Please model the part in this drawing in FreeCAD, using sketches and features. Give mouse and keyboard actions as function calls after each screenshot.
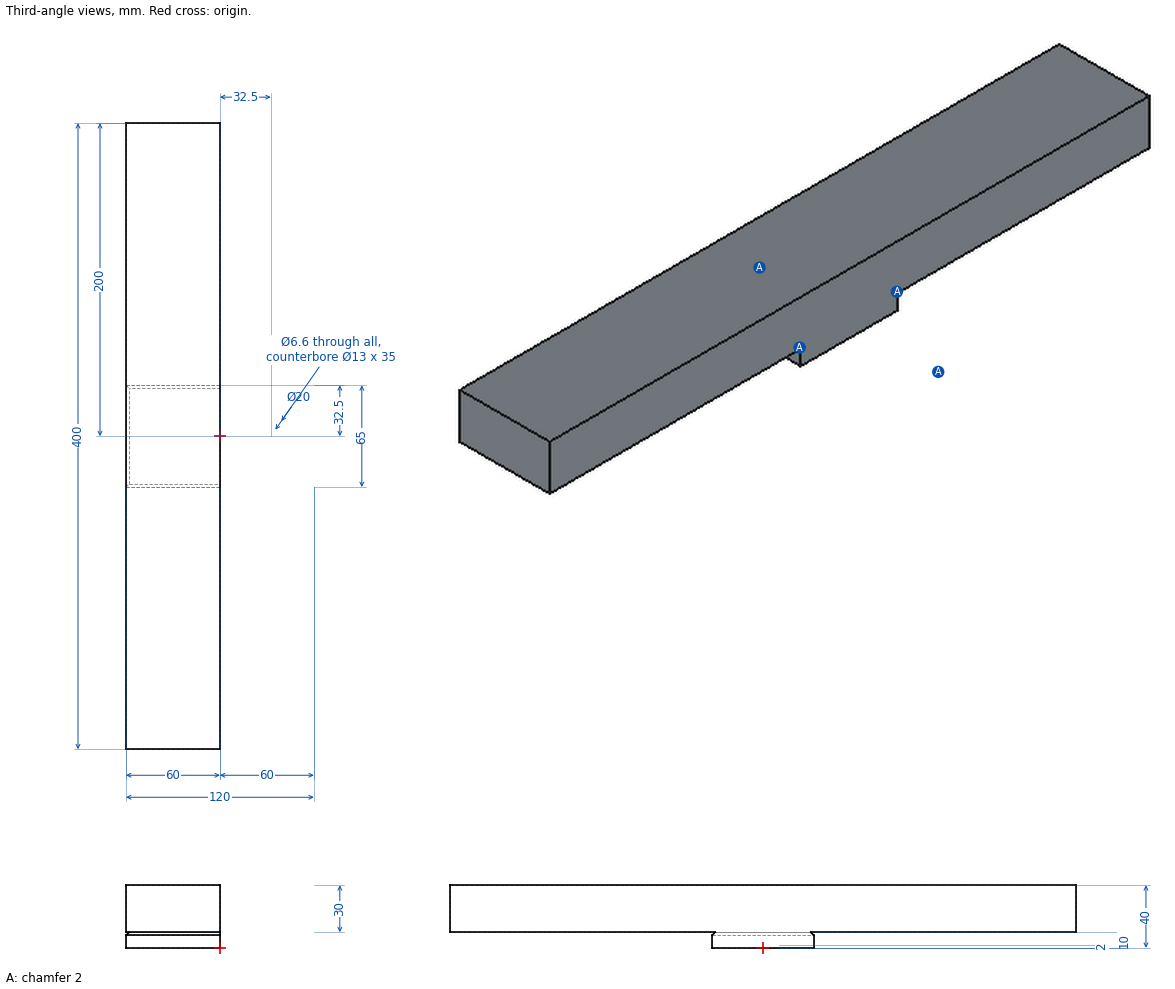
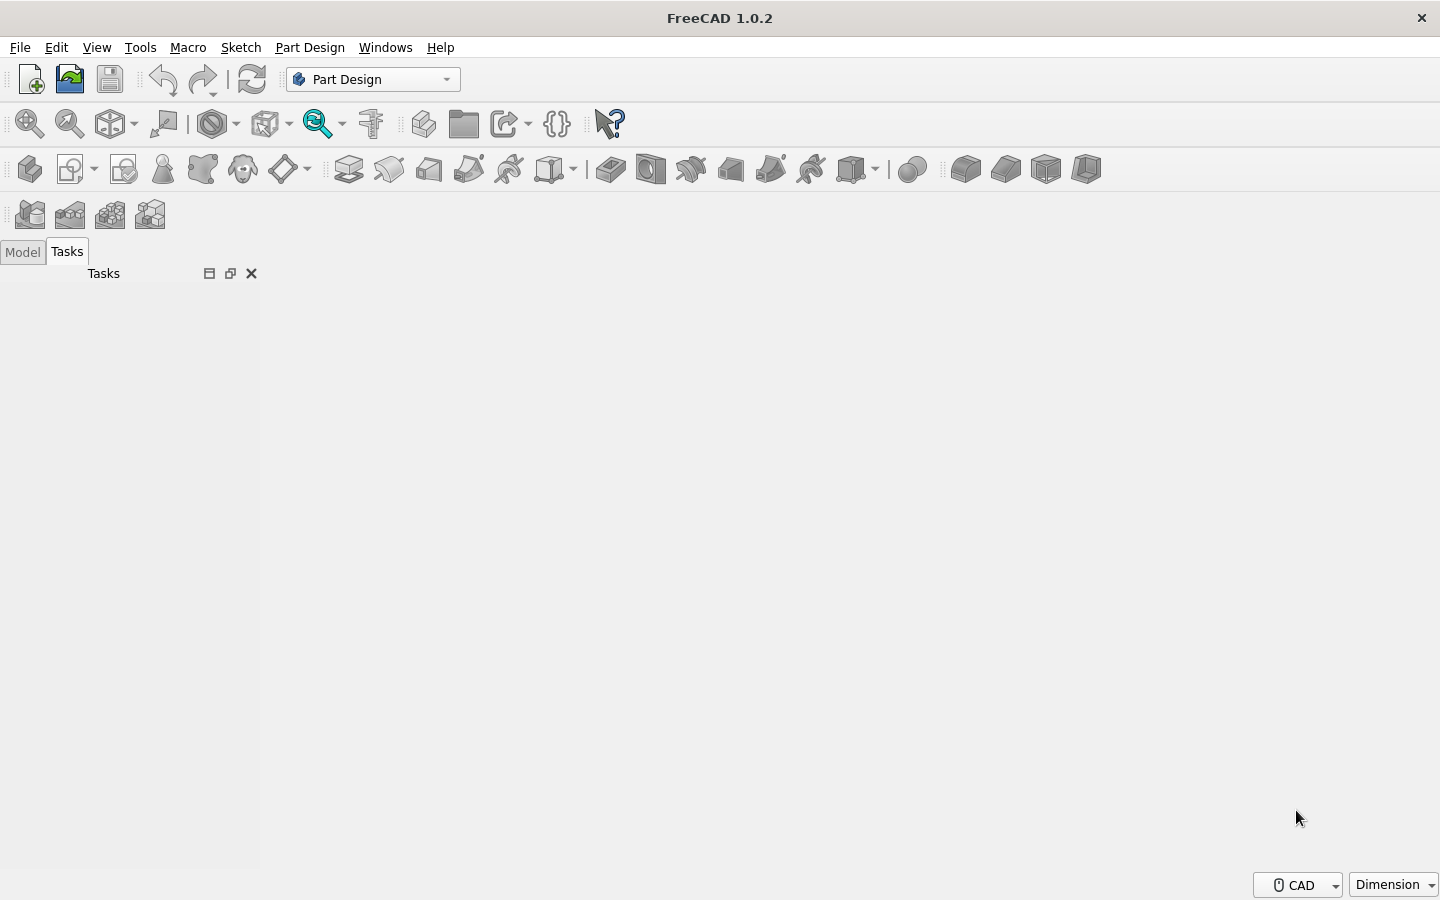
key(ctrl+n)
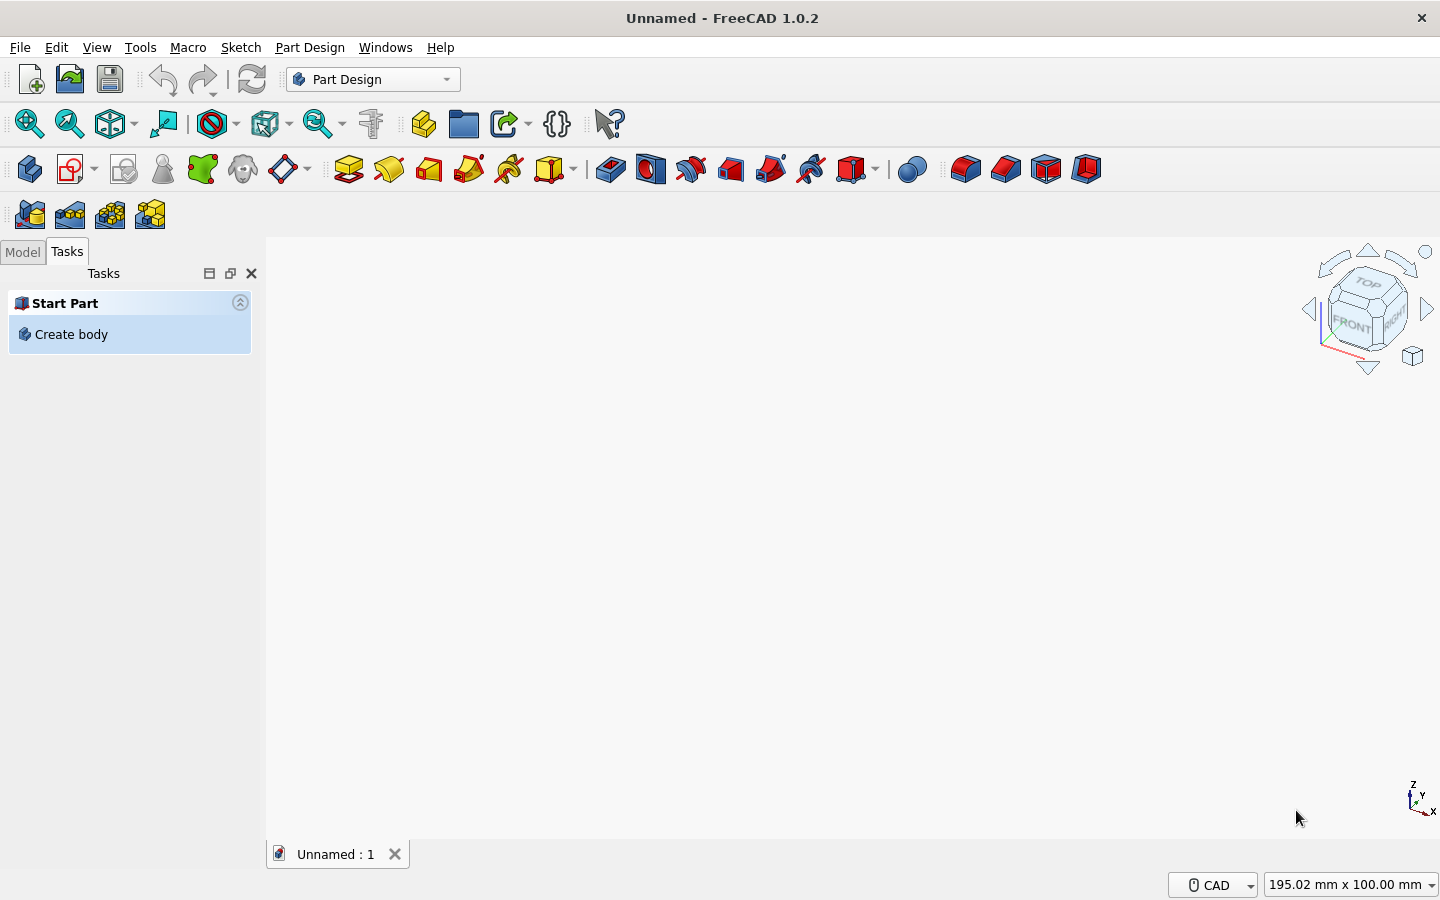
click(70, 170)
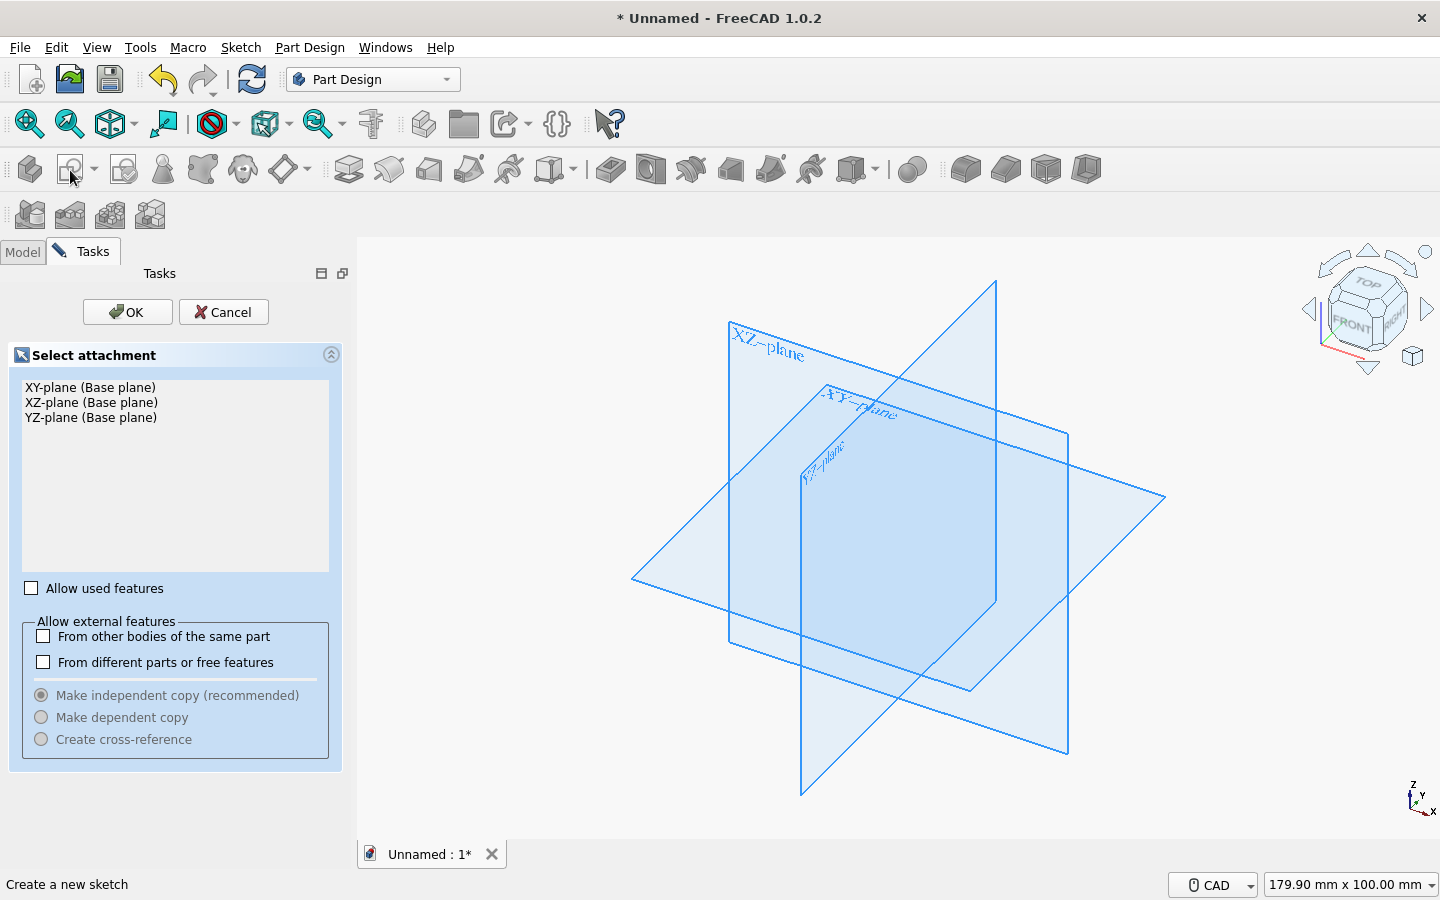
click(82, 388)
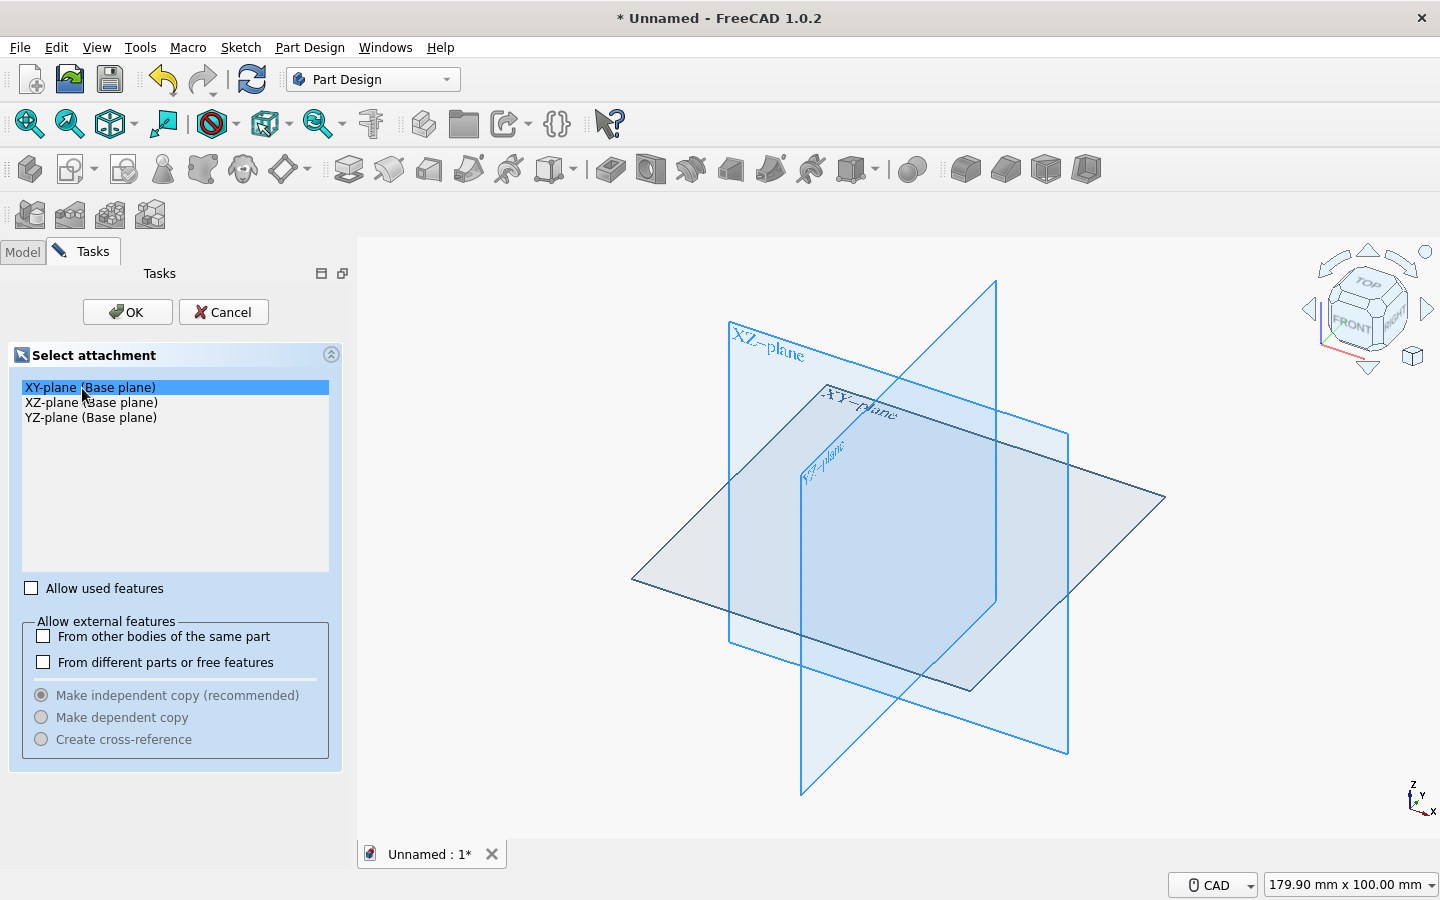
click(128, 312)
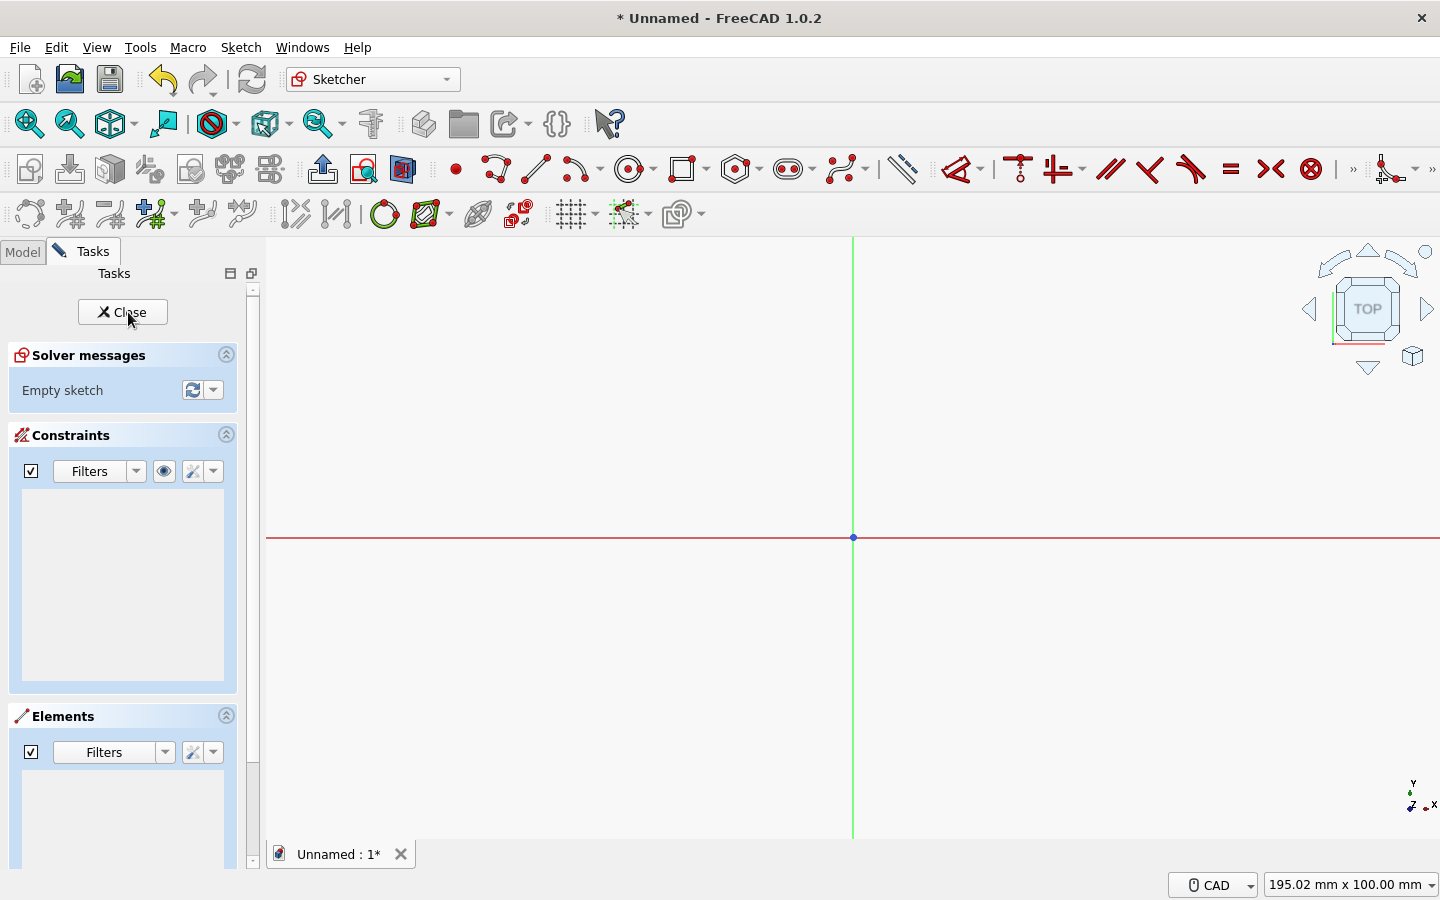
key(g)
key(v)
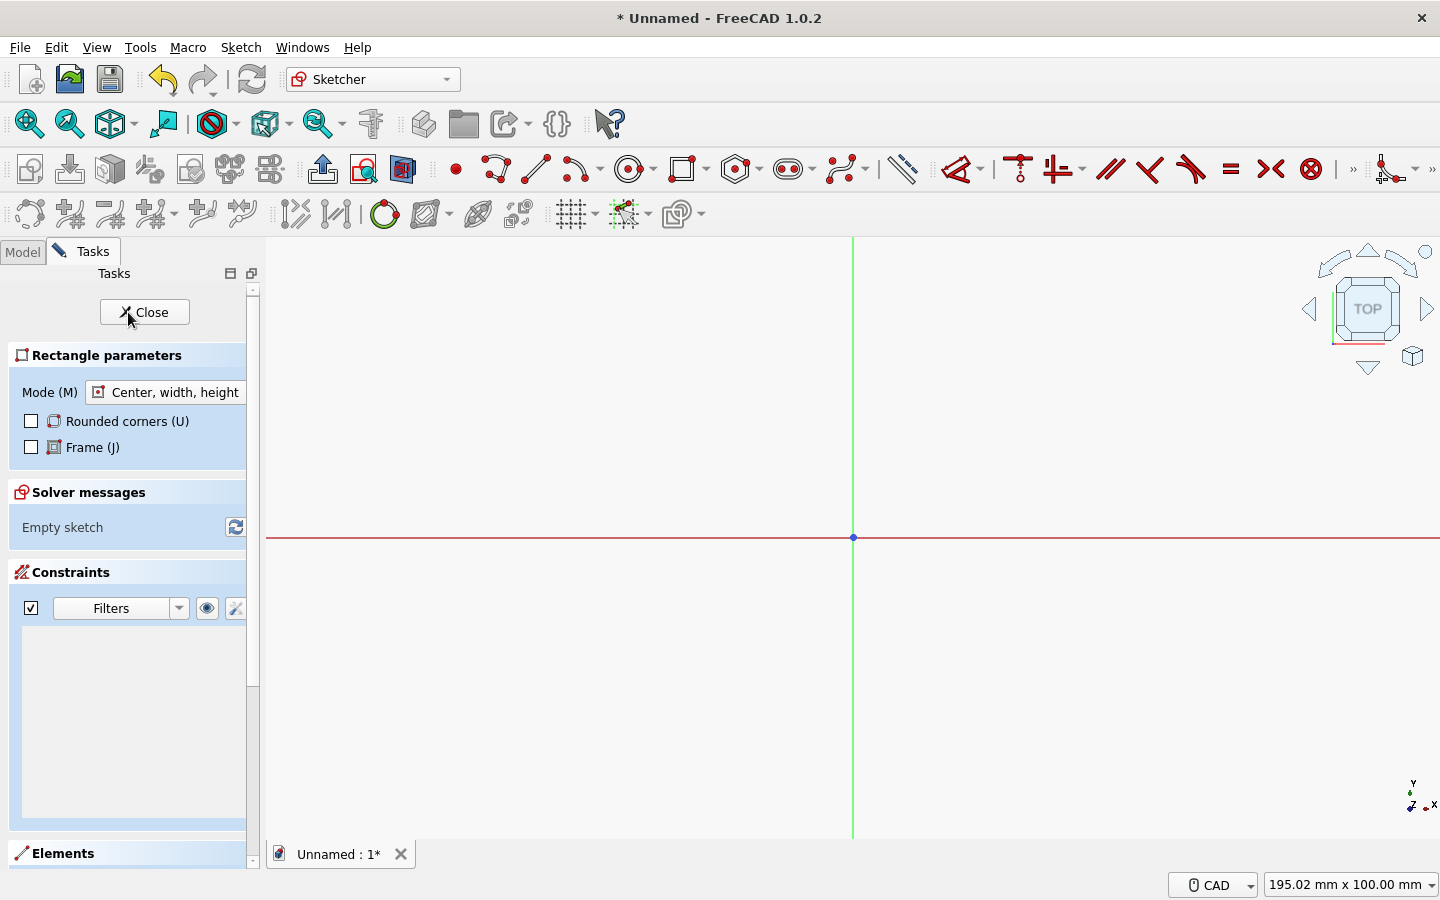
click(853, 538)
click(1214, 342)
key(Escape)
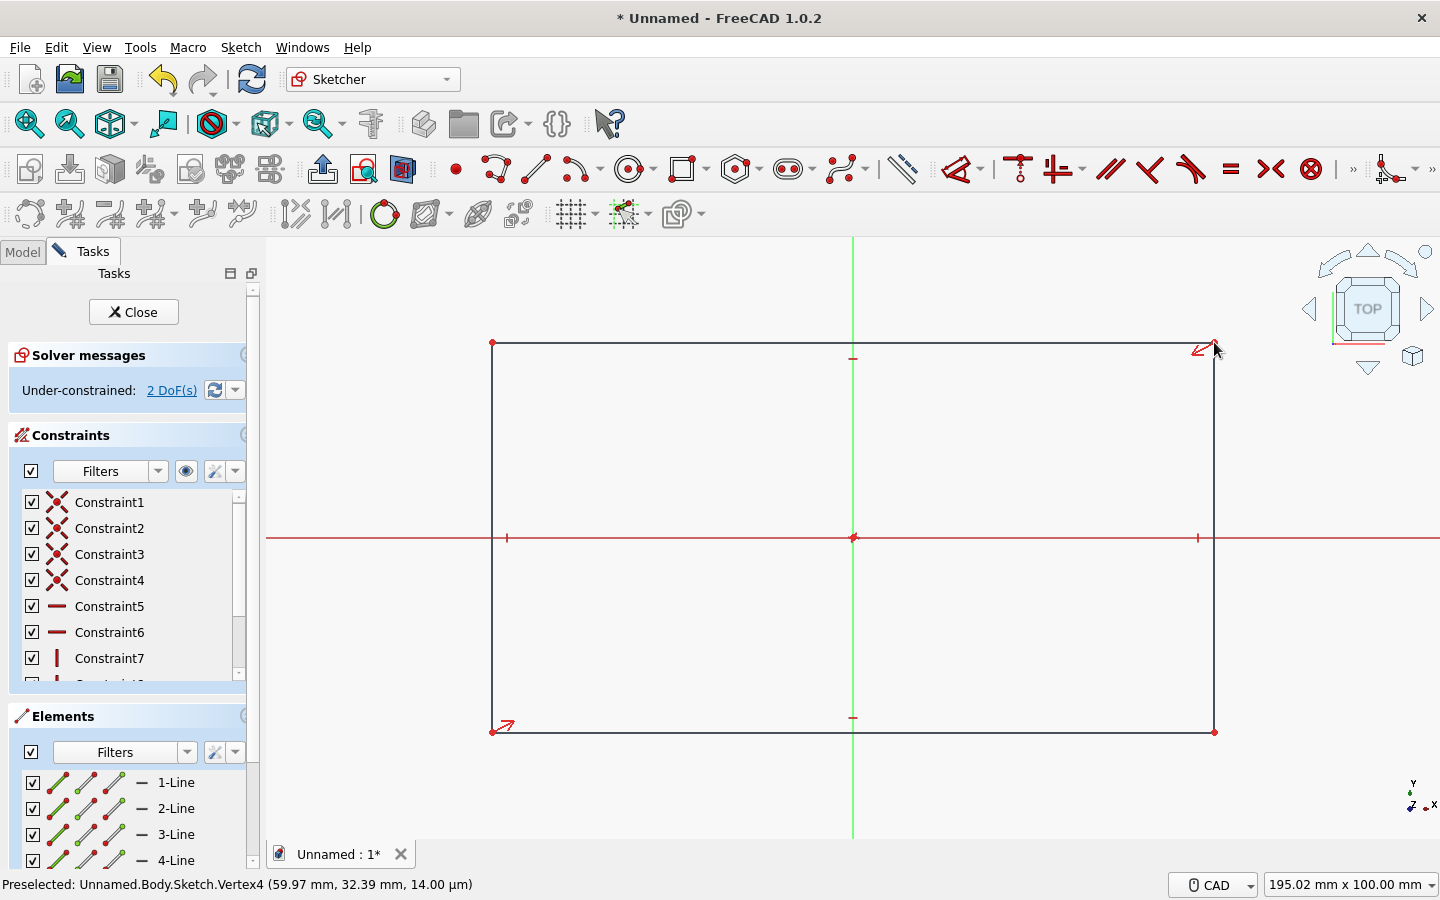
key(d)